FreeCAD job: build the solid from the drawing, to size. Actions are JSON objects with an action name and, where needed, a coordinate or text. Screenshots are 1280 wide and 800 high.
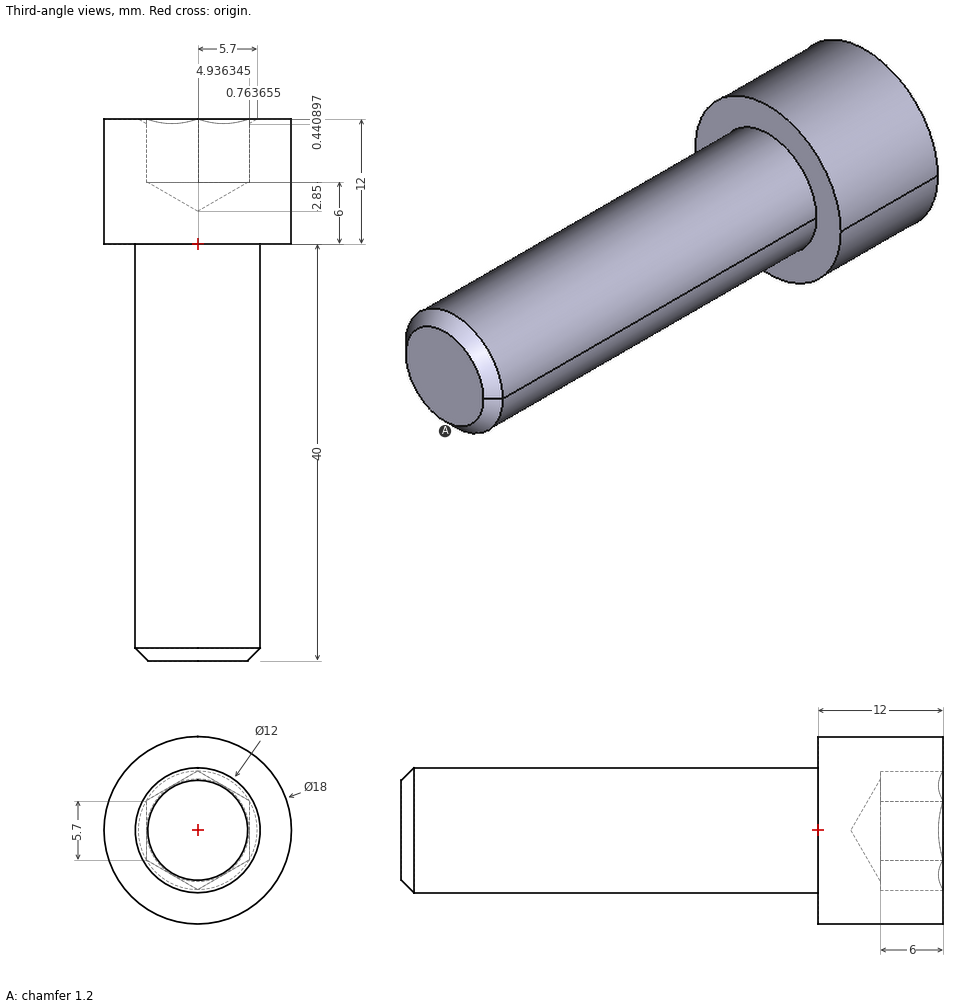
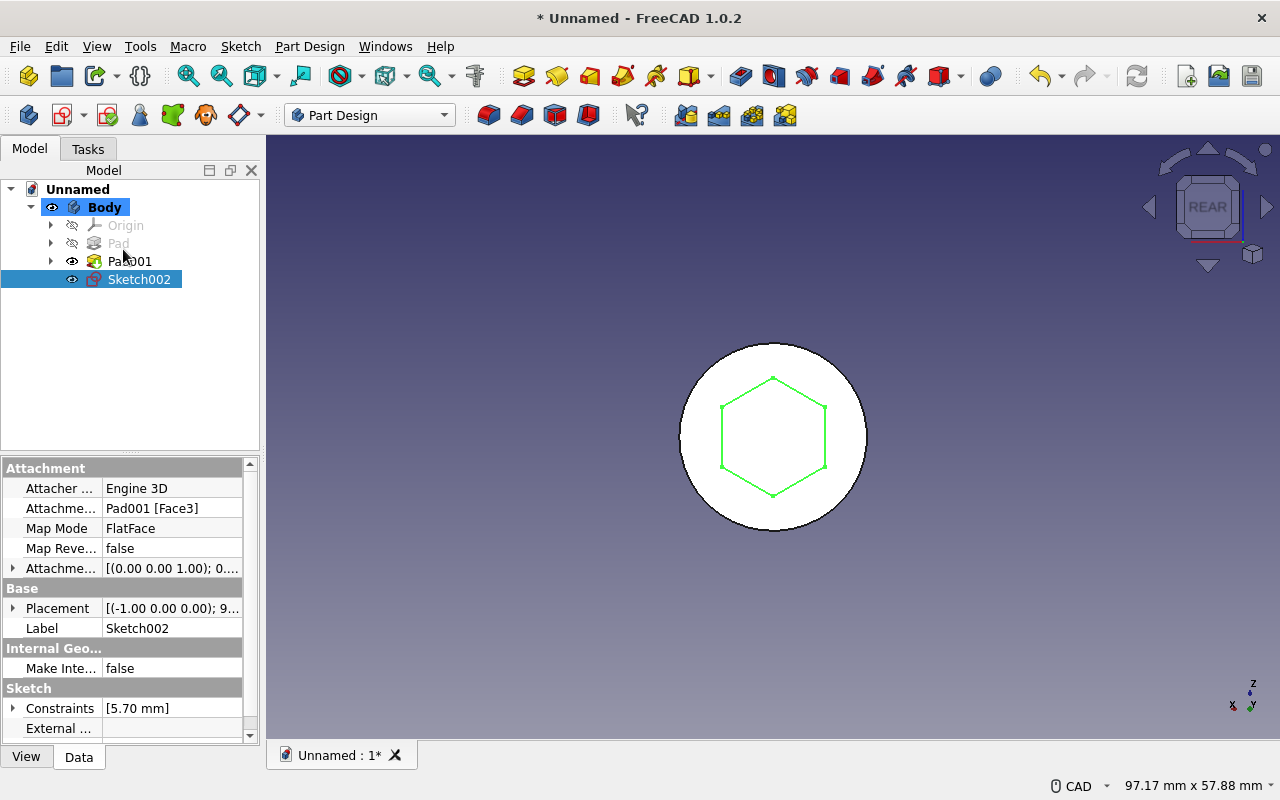
{"action": "left_click", "coordinate": [741, 76]}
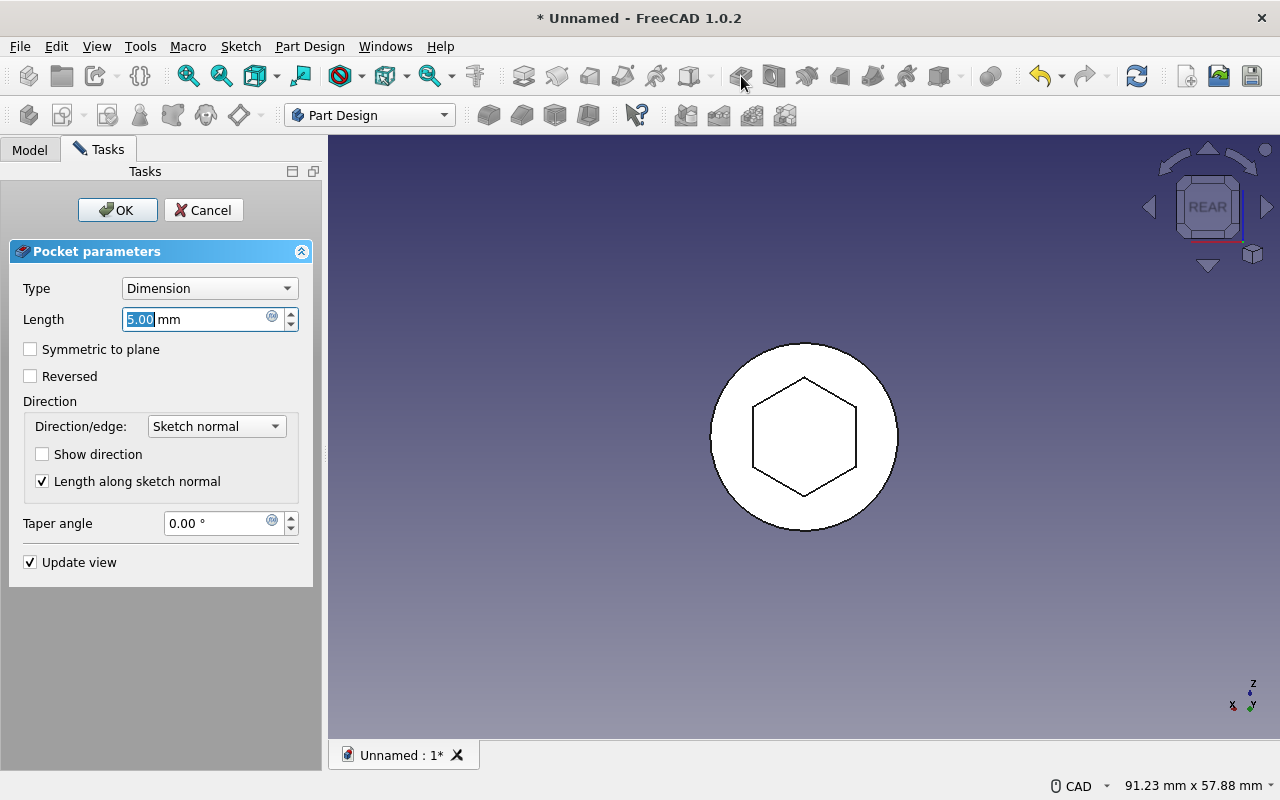
{"action": "type", "text": "6"}
{"action": "key", "text": "Tab"}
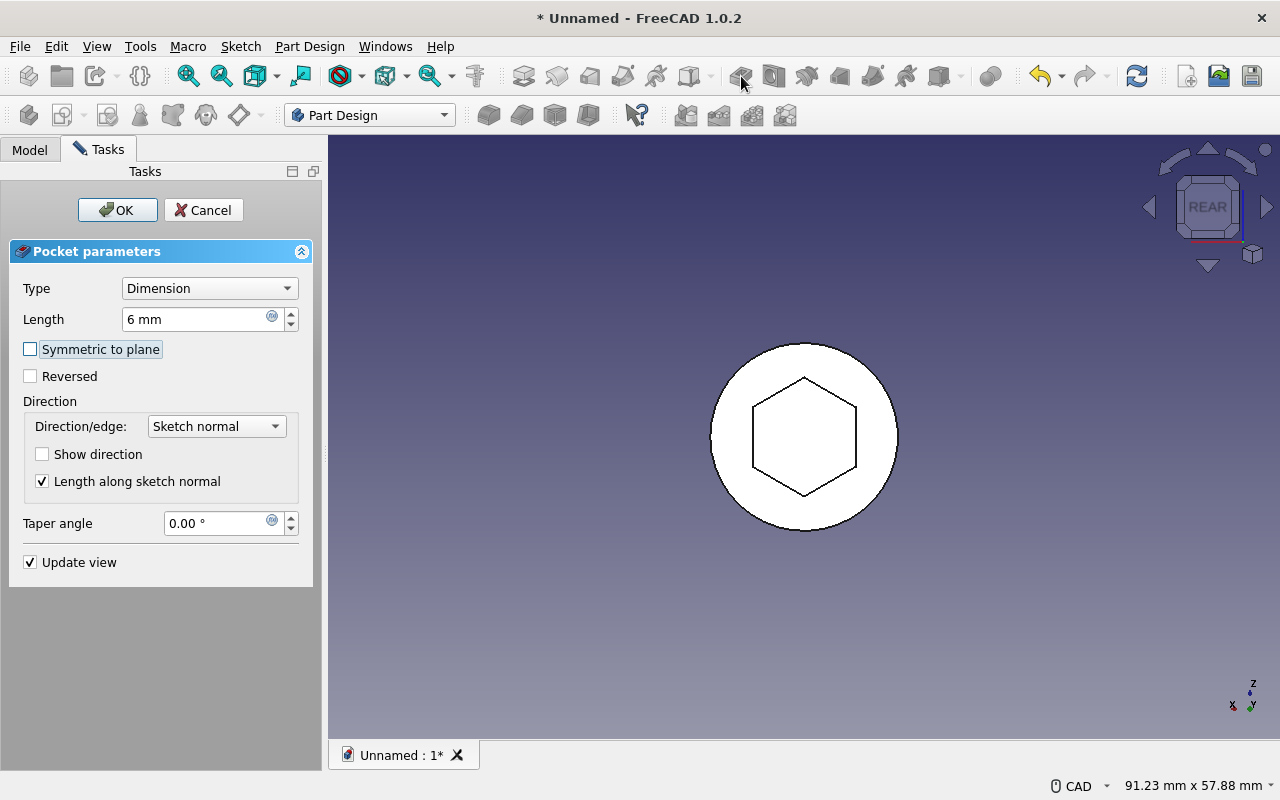
{"action": "left_click", "coordinate": [118, 210]}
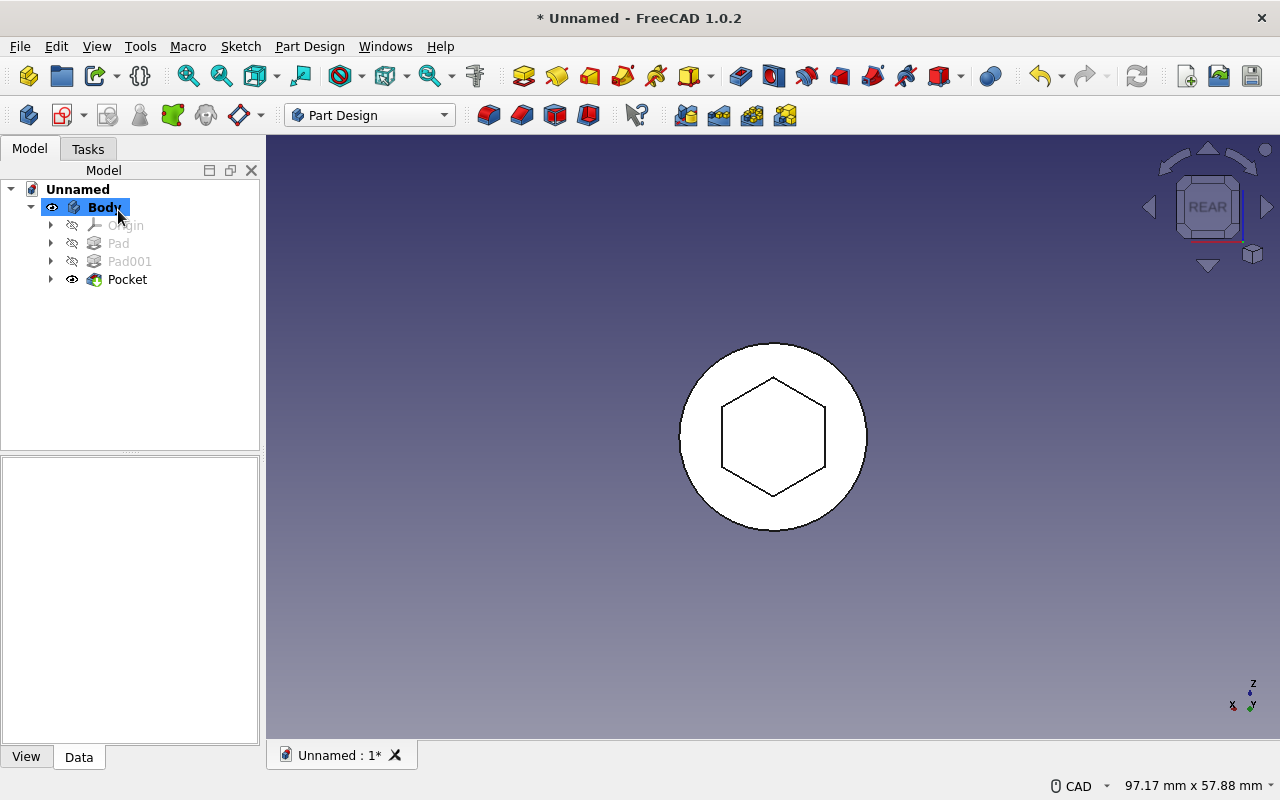
{"action": "left_click", "coordinate": [189, 76]}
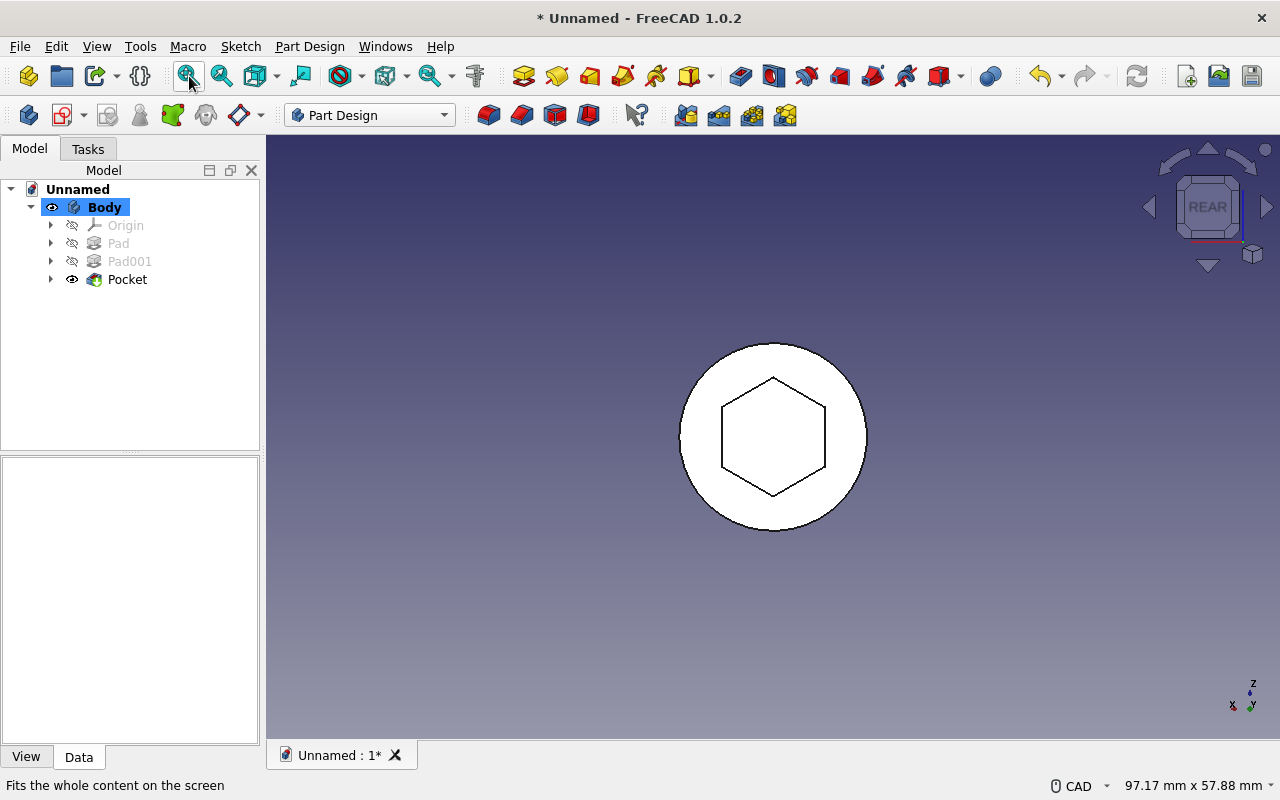
{"action": "left_click", "coordinate": [62, 116]}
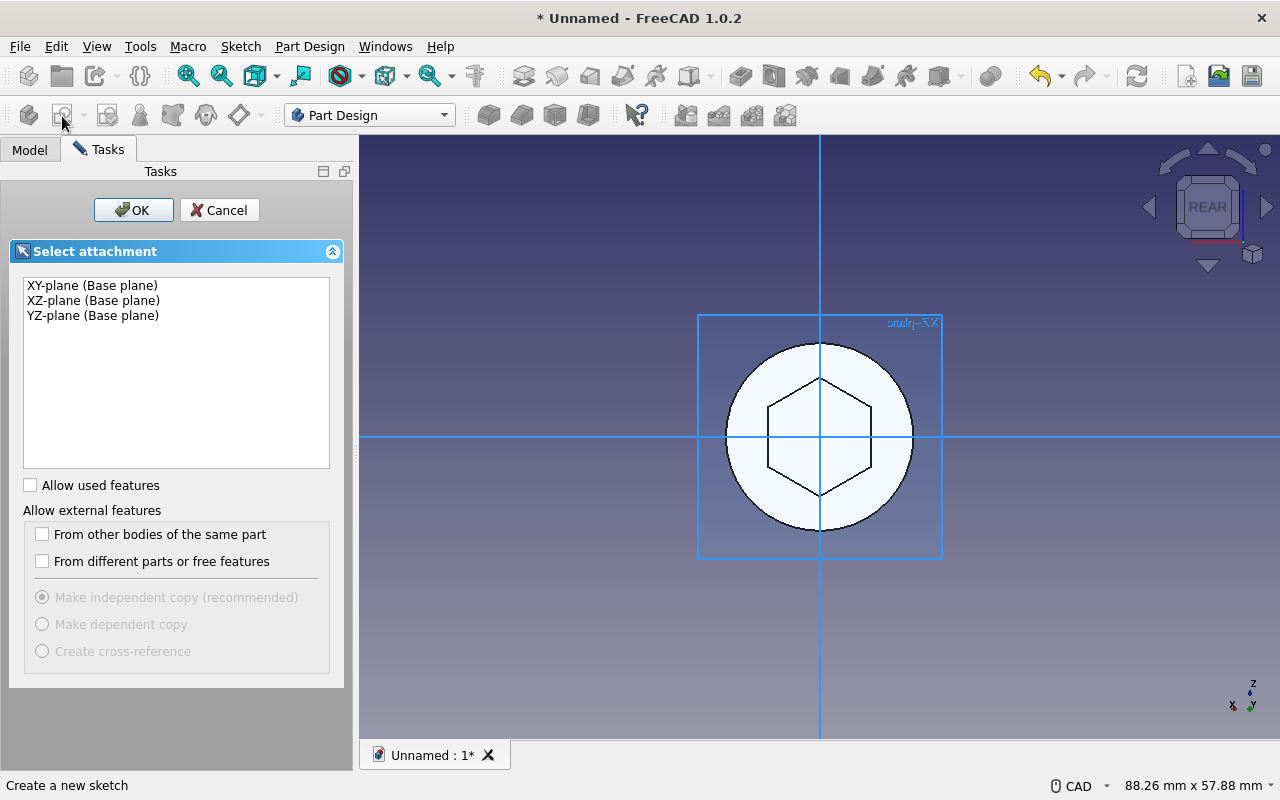
{"action": "left_click", "coordinate": [84, 286]}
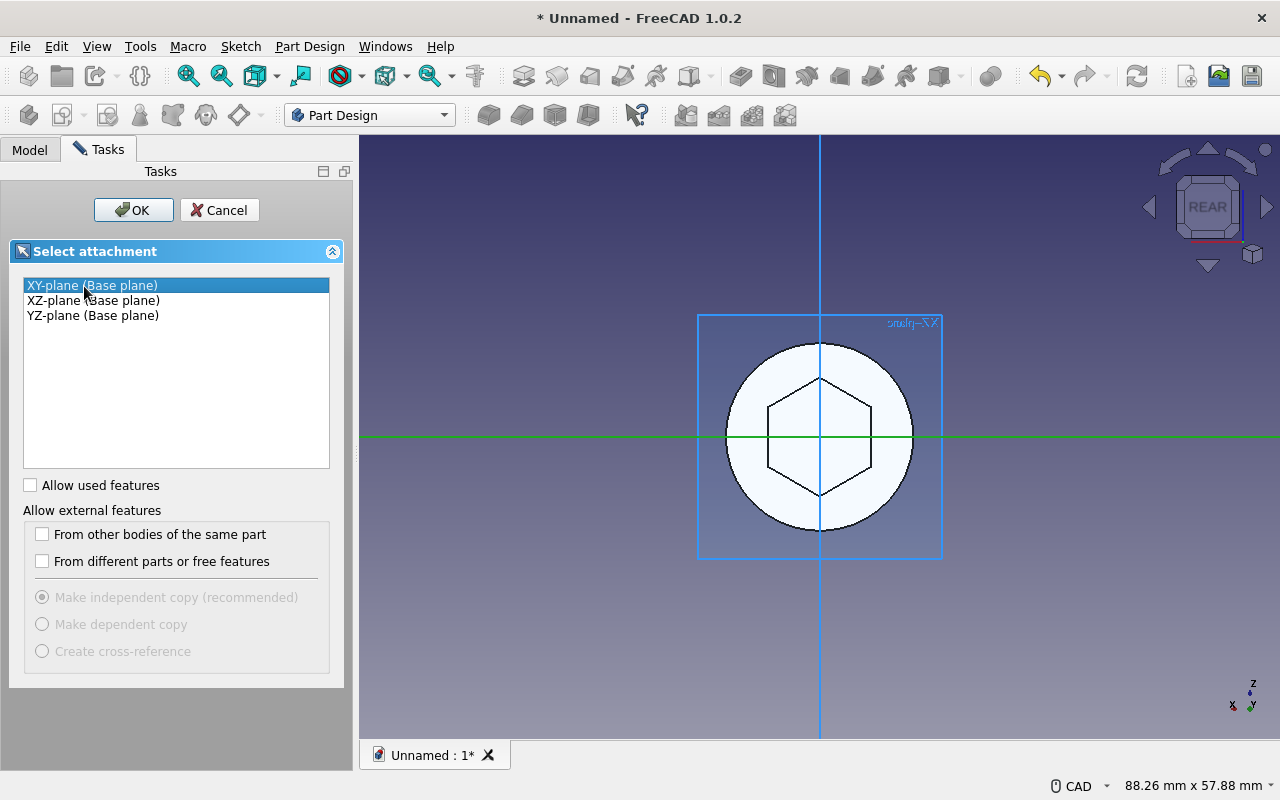
{"action": "left_click", "coordinate": [134, 210]}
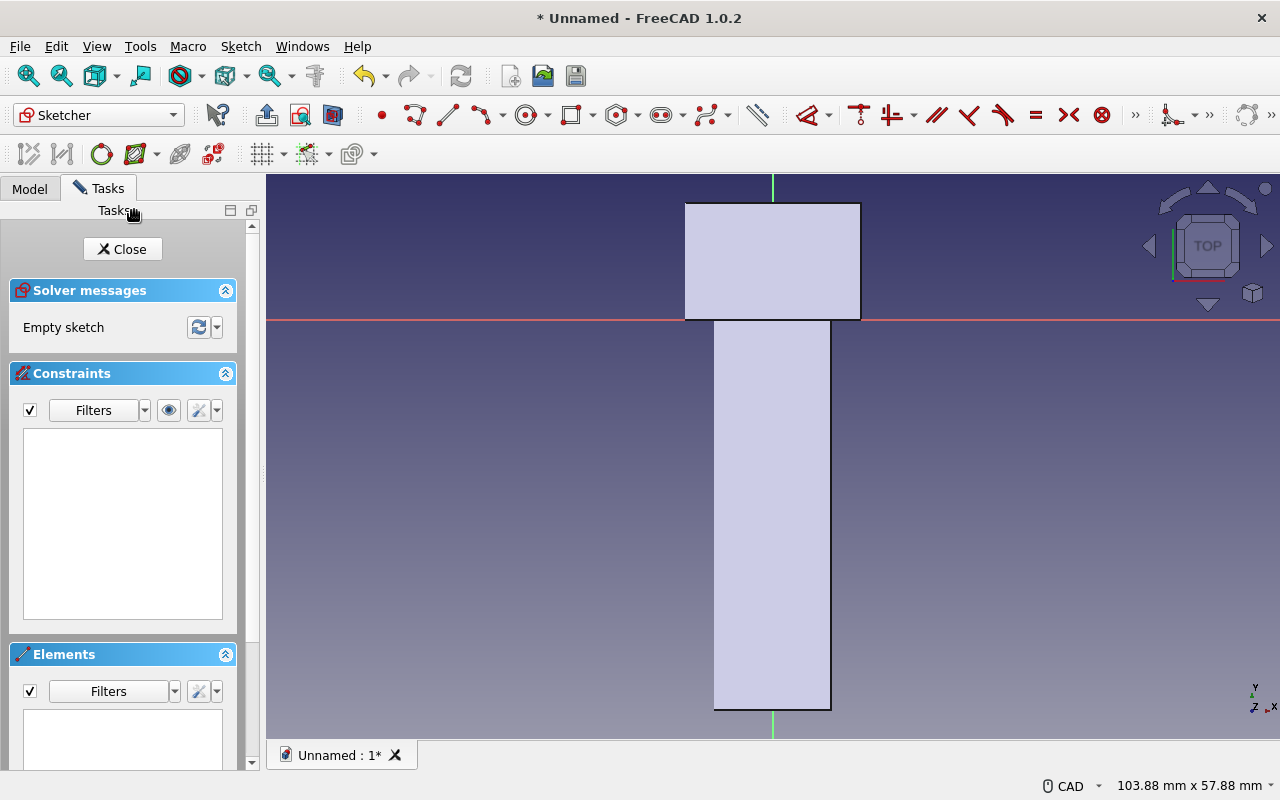
{"action": "left_click", "coordinate": [333, 116]}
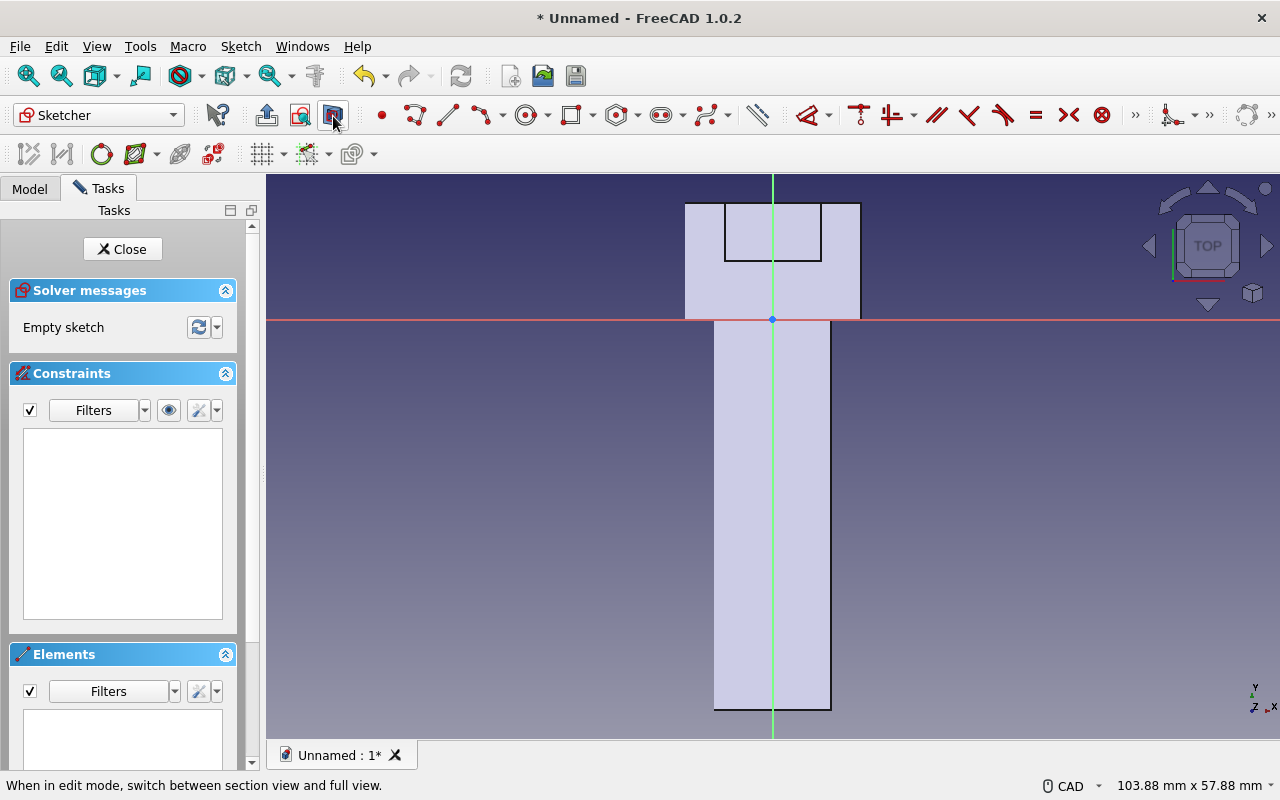
{"action": "scroll", "coordinate": [704, 456], "scroll_direction": "down", "scroll_amount": 5}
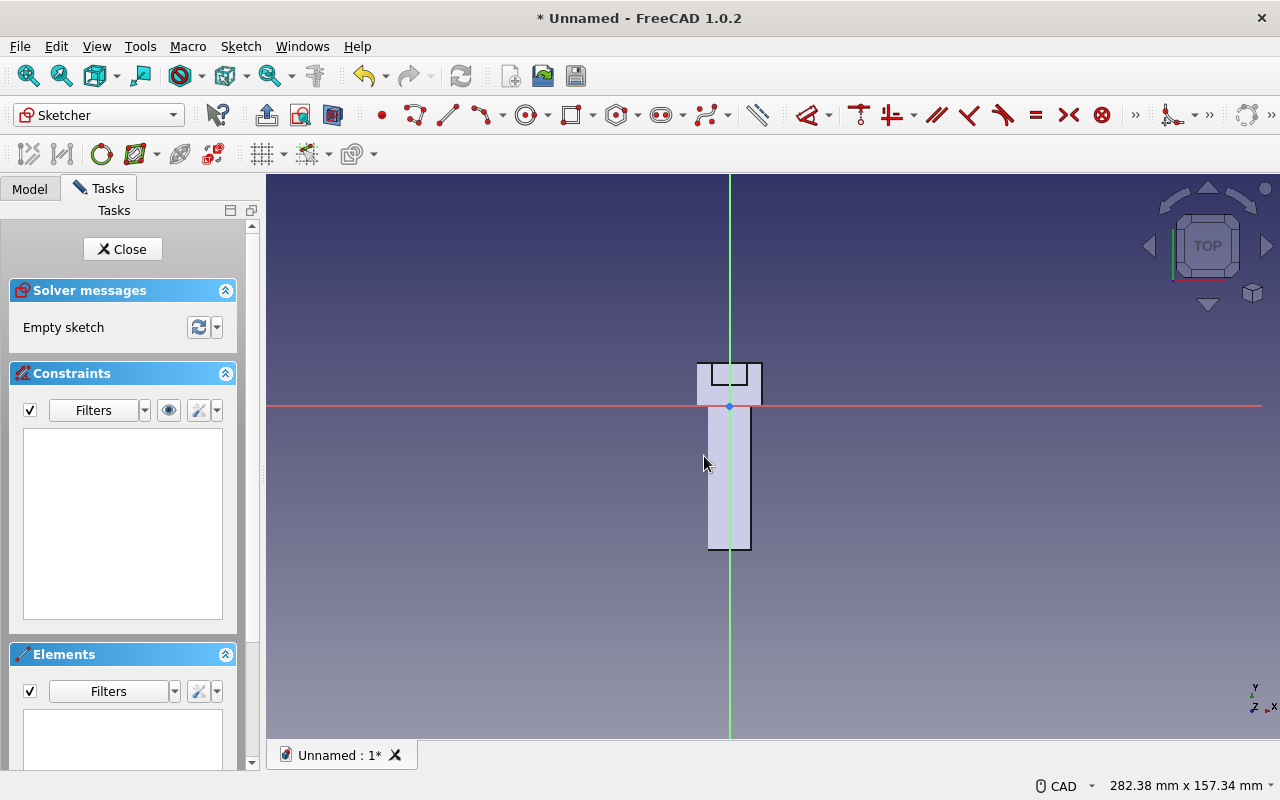
{"action": "scroll", "coordinate": [744, 376], "scroll_direction": "up", "scroll_amount": 11}